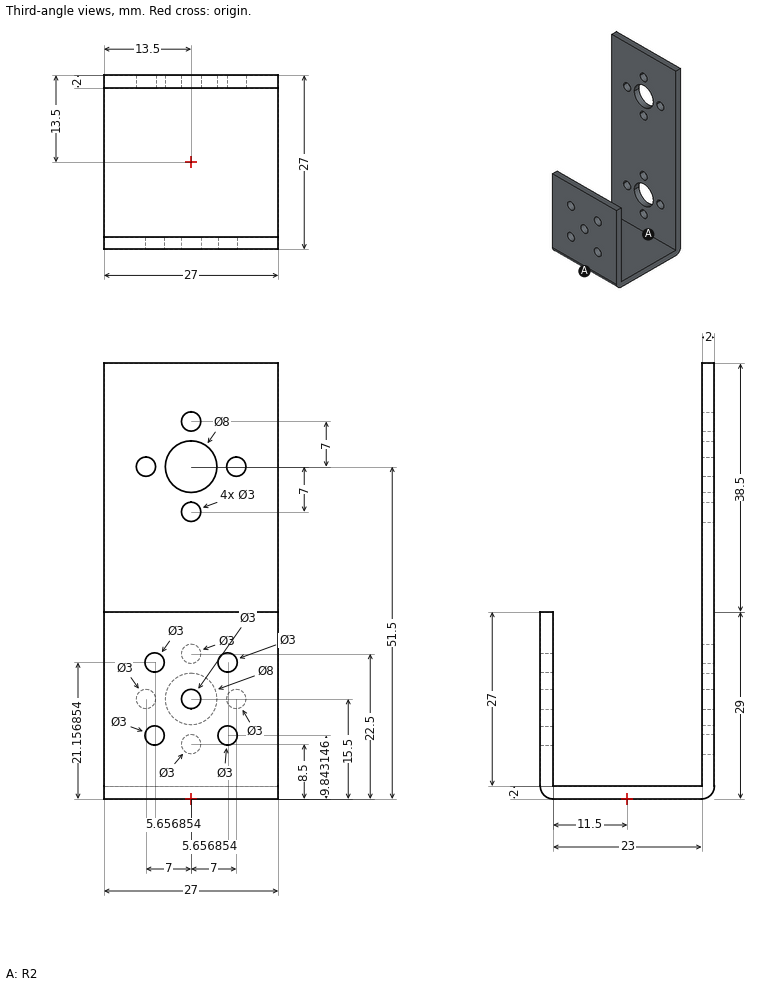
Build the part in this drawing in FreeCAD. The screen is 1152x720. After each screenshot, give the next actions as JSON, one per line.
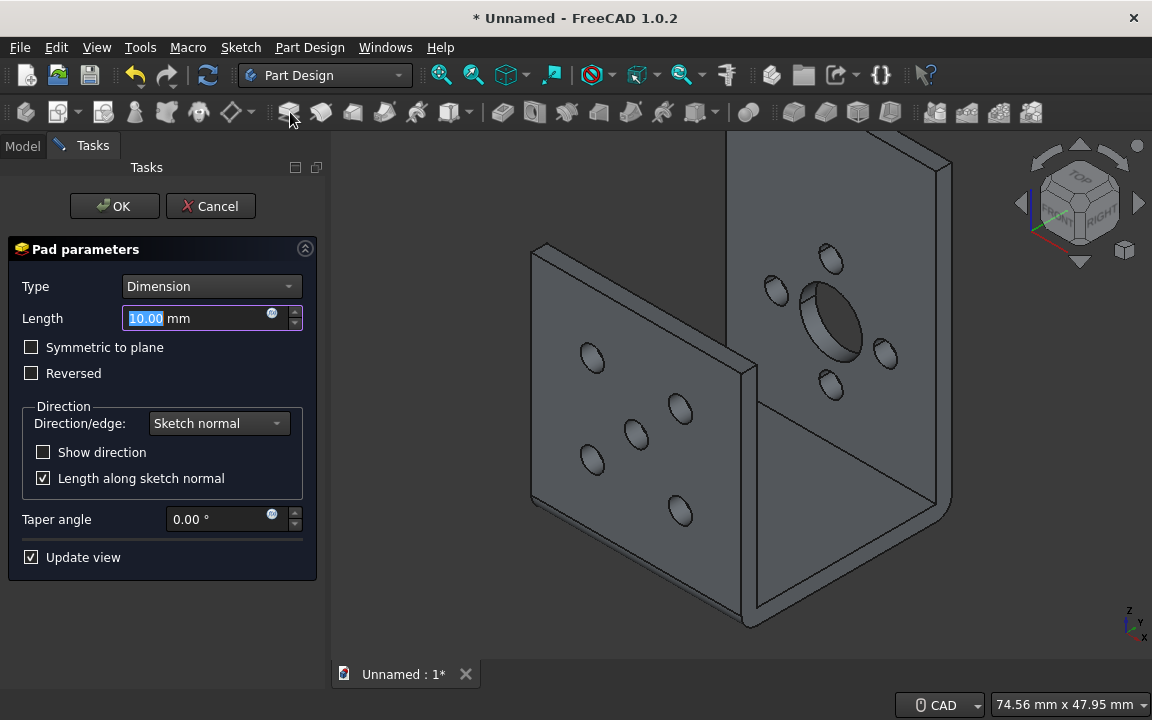
{"action": "type", "text": "38.5"}
{"action": "key", "text": "Tab"}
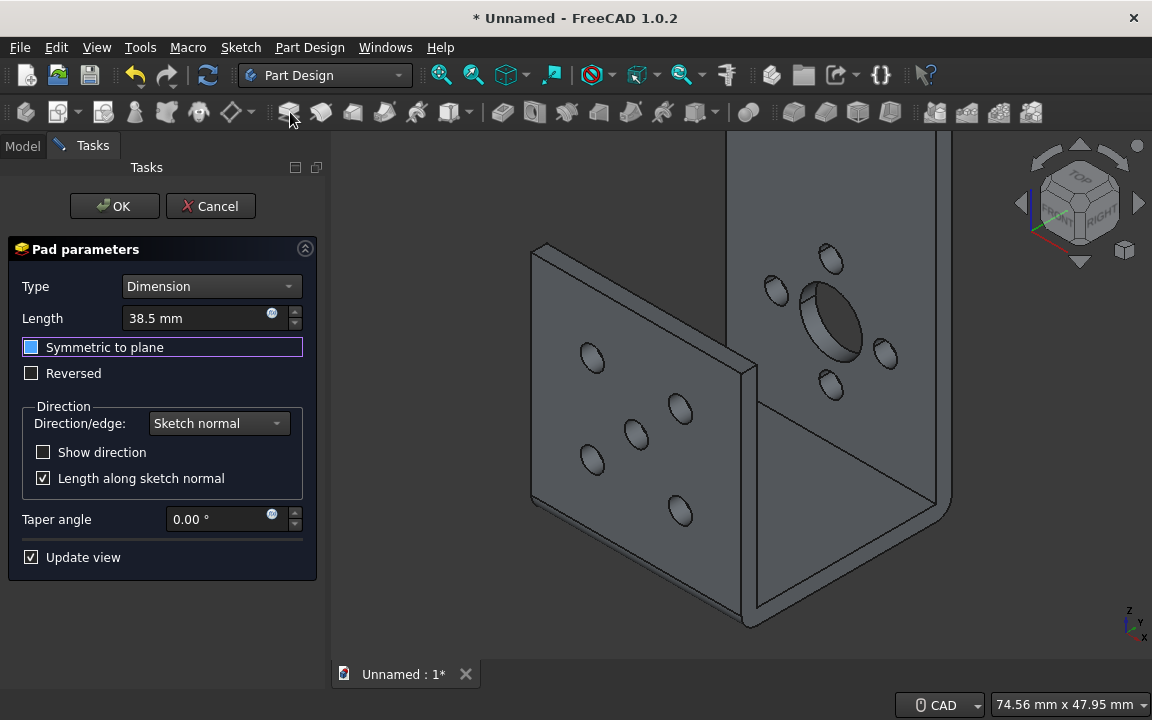
{"action": "left_click", "coordinate": [115, 206]}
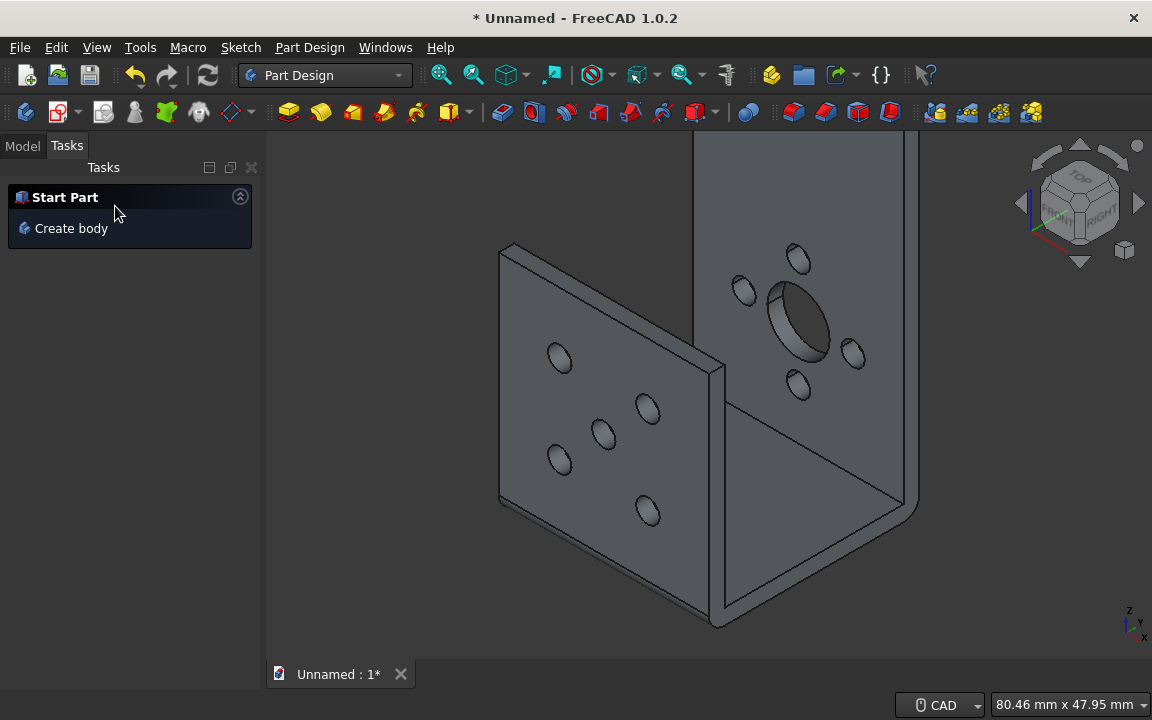
{"action": "left_click", "coordinate": [442, 76]}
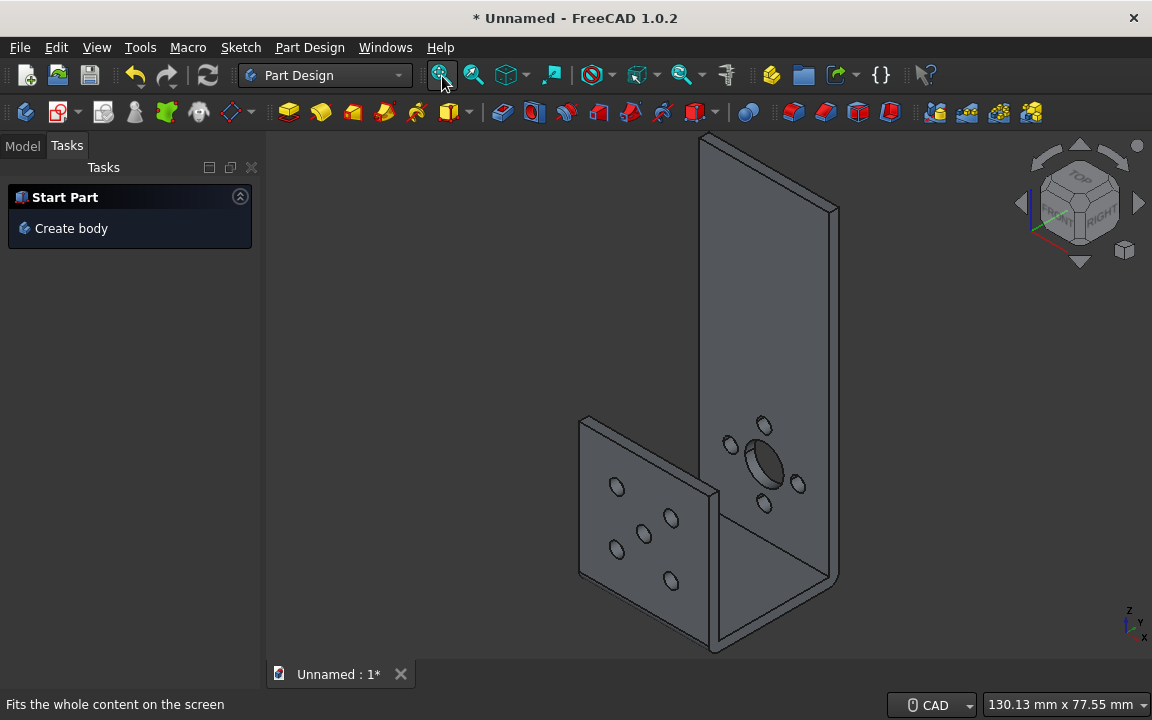
{"action": "key", "text": "4"}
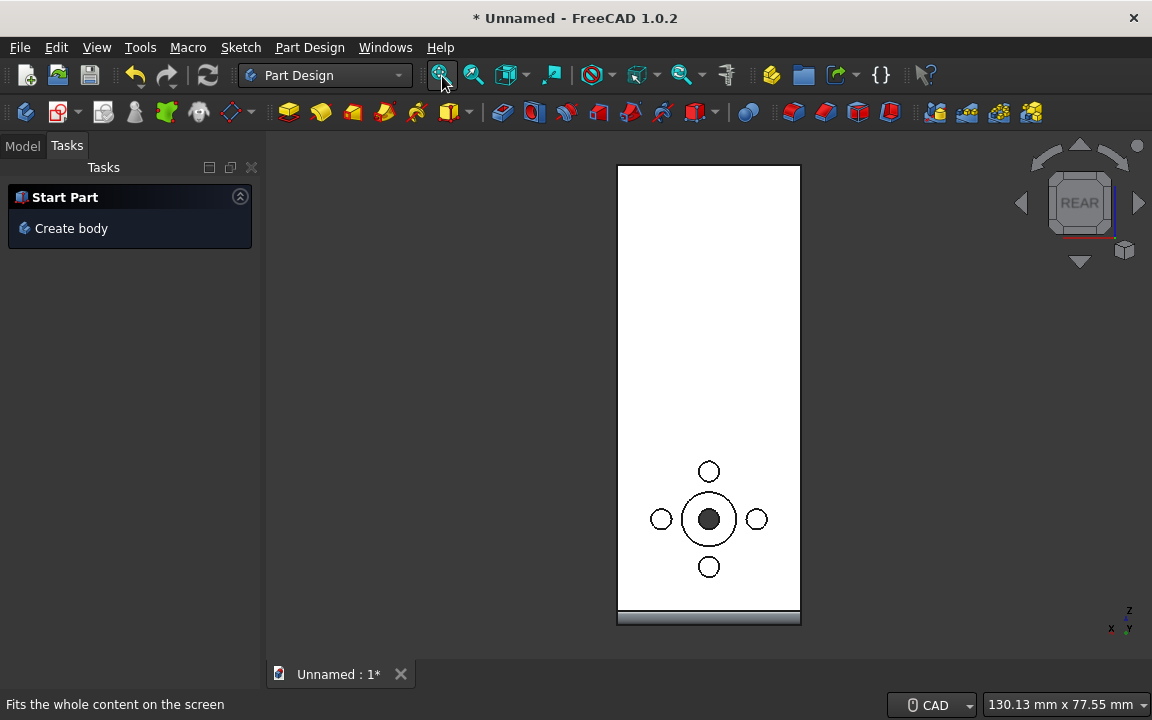
{"action": "left_click", "coordinate": [709, 260]}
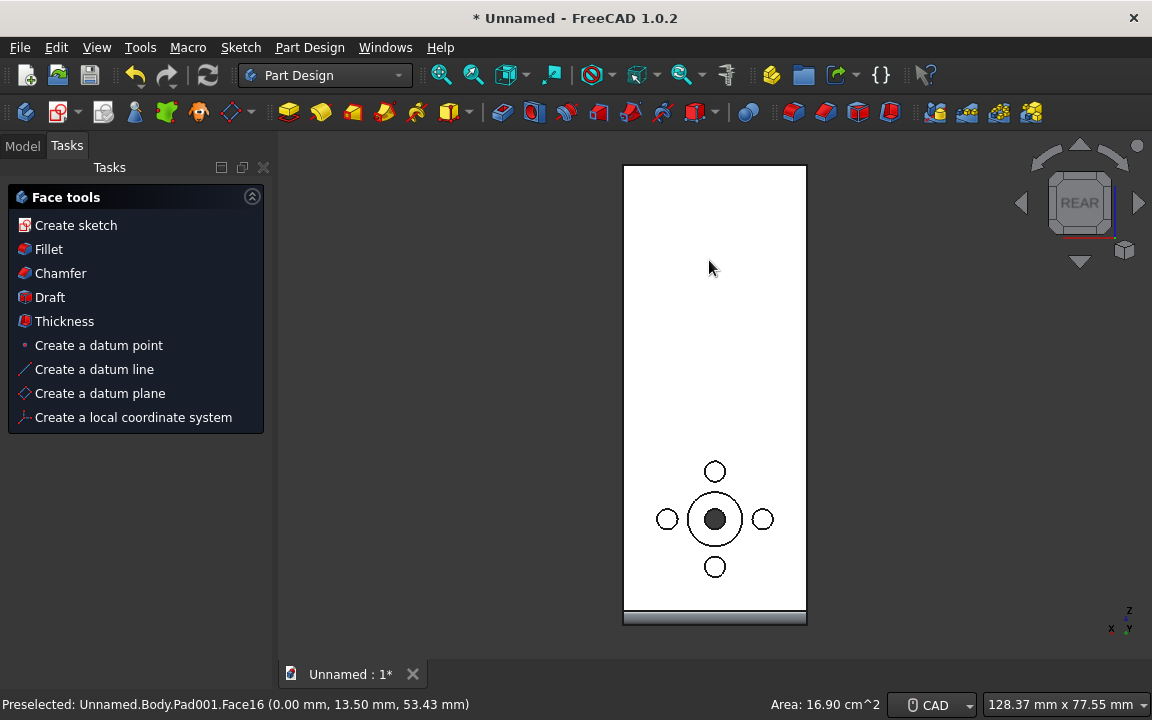
{"action": "left_click", "coordinate": [58, 112]}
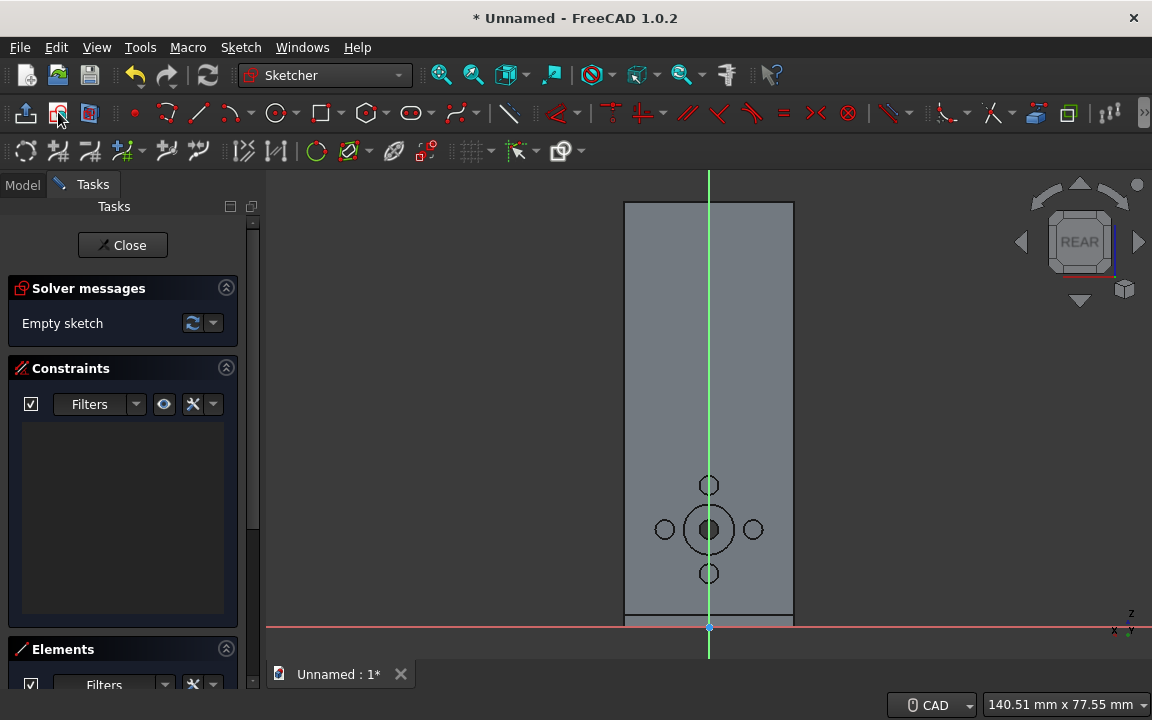
{"action": "scroll", "coordinate": [749, 237], "scroll_direction": "up", "scroll_amount": 5}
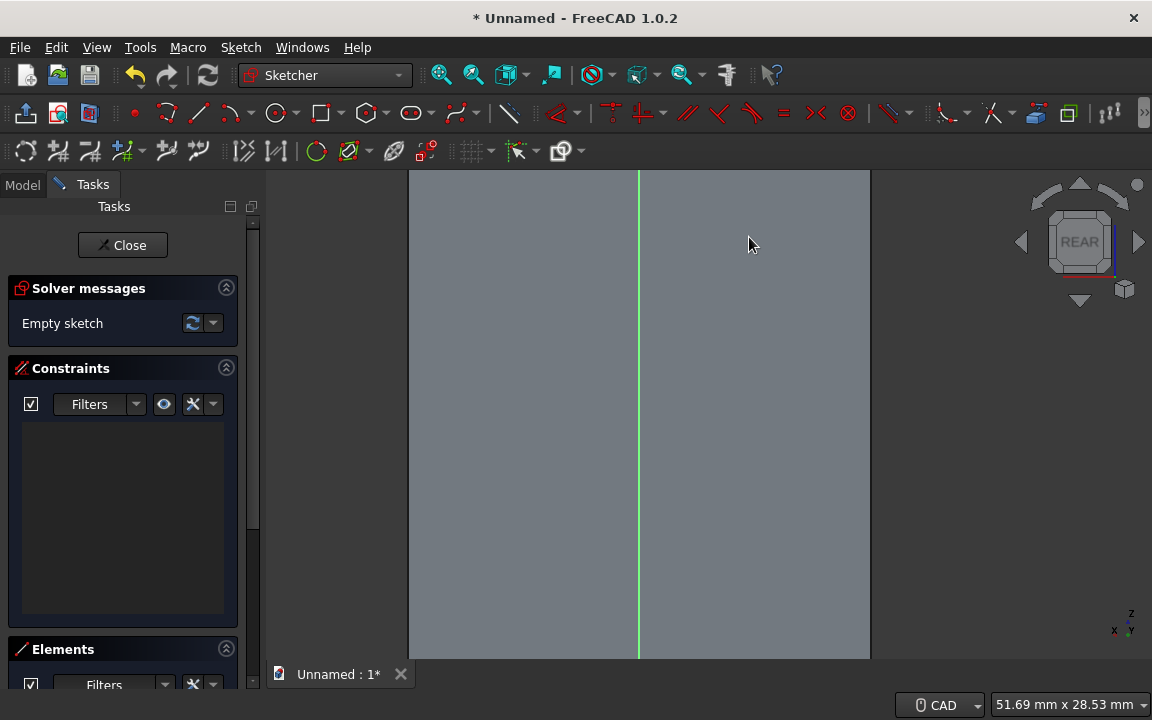
{"action": "key", "text": "g c"}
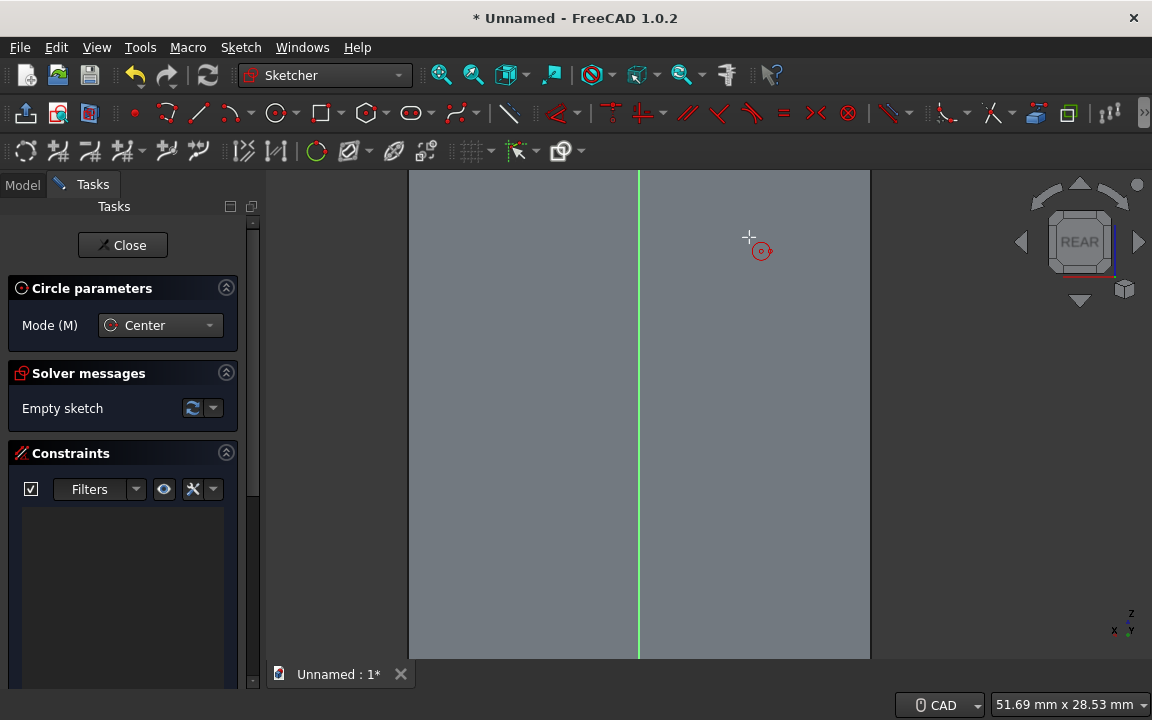
{"action": "left_click", "coordinate": [639, 415]}
{"action": "left_click", "coordinate": [688, 367]}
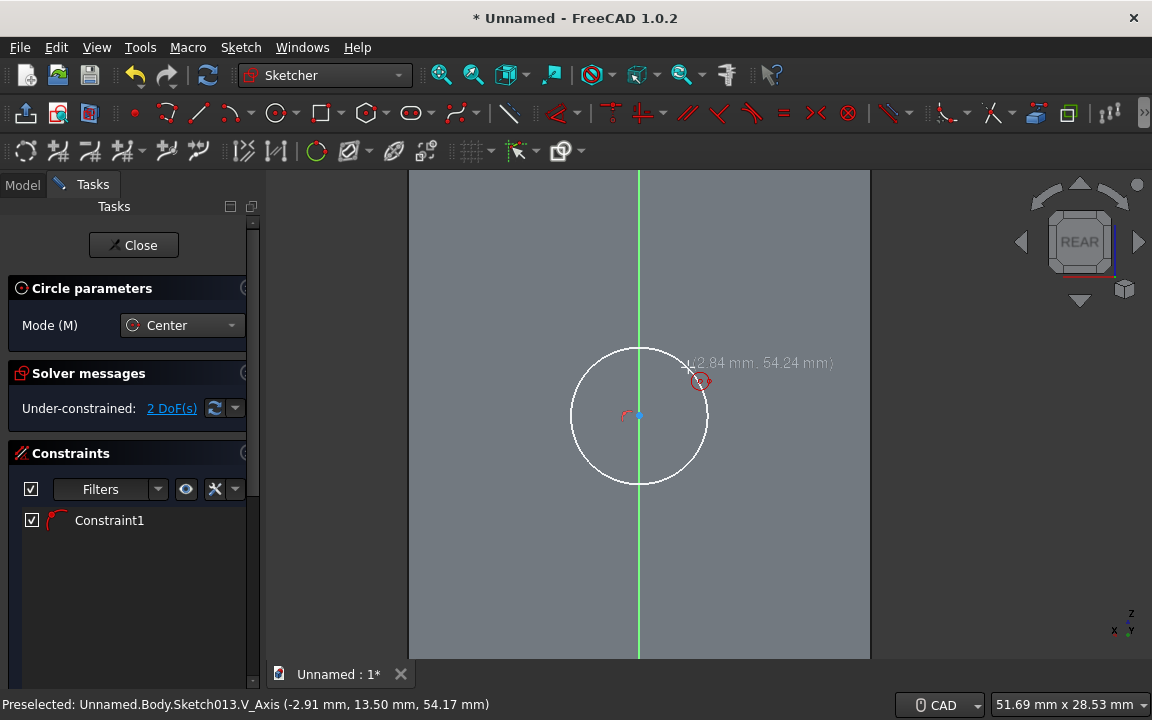
{"action": "left_click", "coordinate": [639, 535]}
{"action": "left_click", "coordinate": [658, 517]}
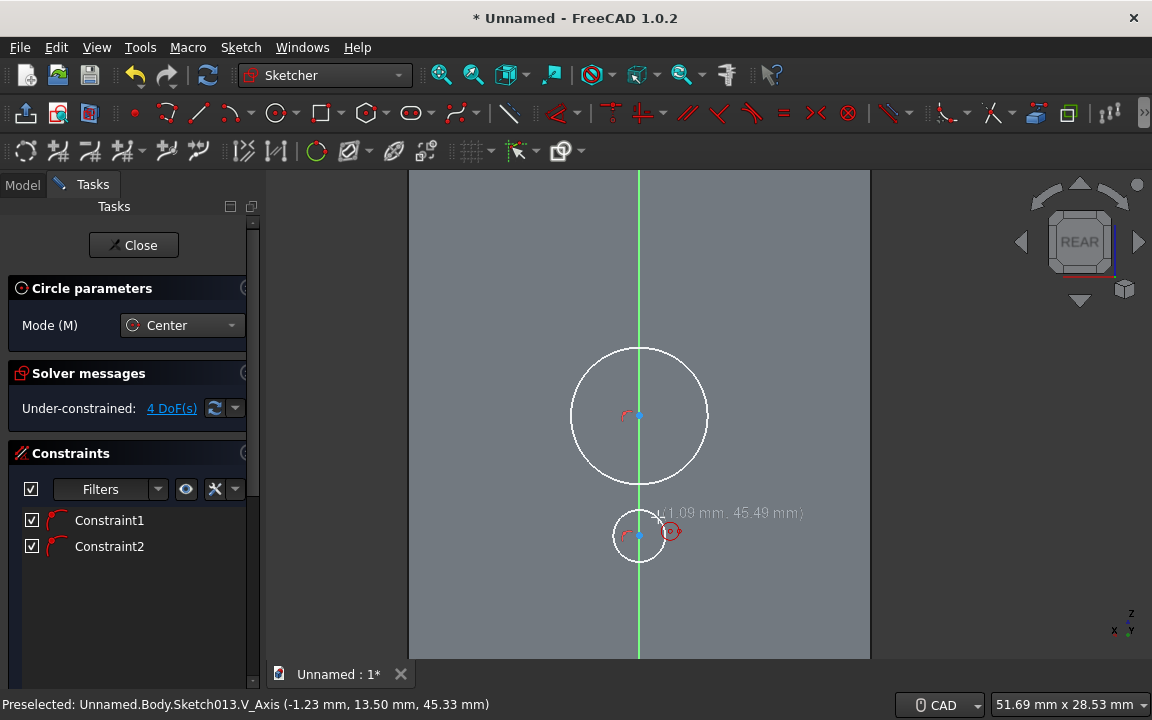
{"action": "left_click", "coordinate": [519, 415]}
{"action": "left_click", "coordinate": [538, 397]}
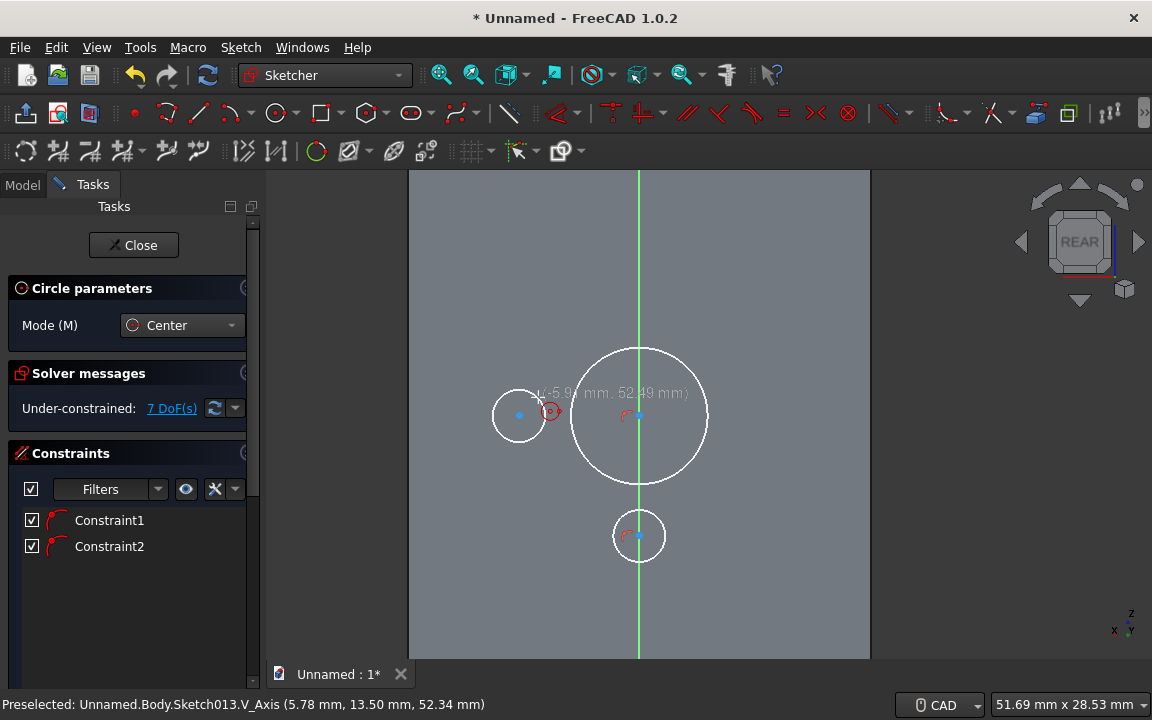
{"action": "left_click", "coordinate": [639, 295]}
{"action": "left_click", "coordinate": [658, 277]}